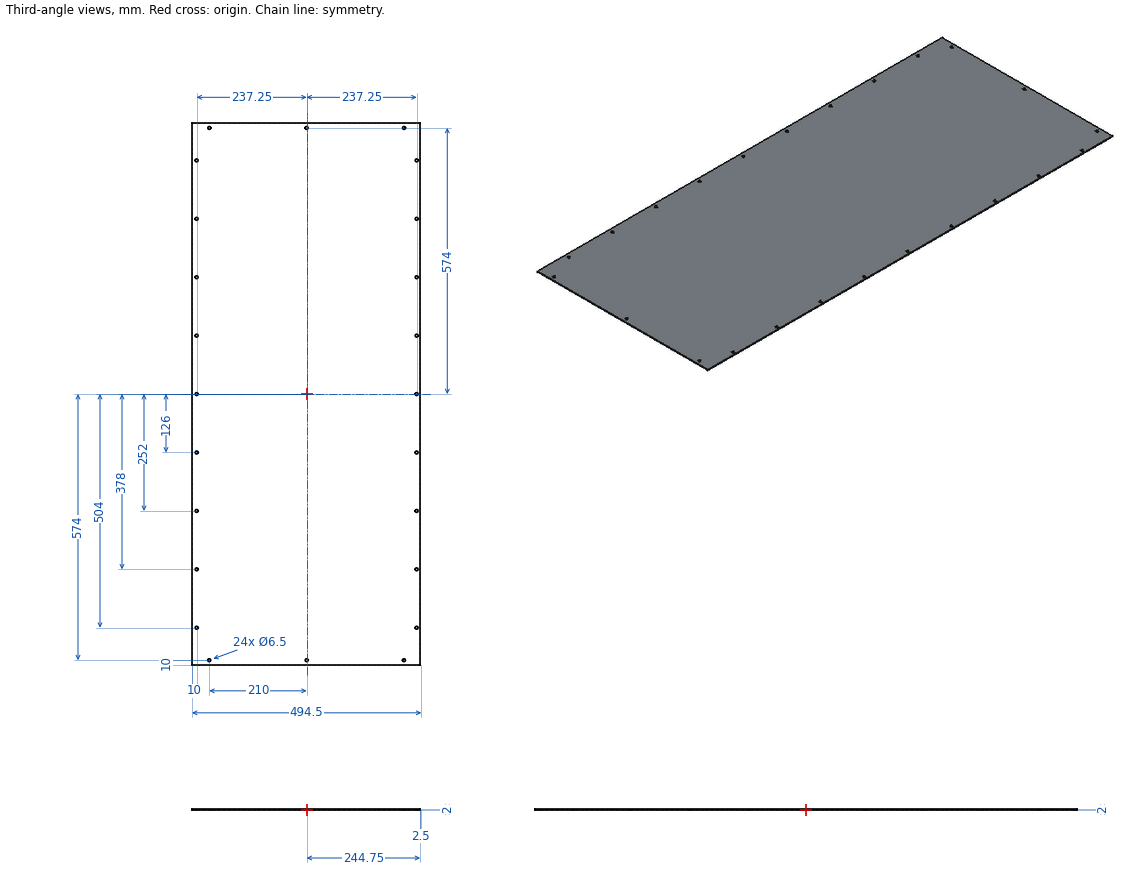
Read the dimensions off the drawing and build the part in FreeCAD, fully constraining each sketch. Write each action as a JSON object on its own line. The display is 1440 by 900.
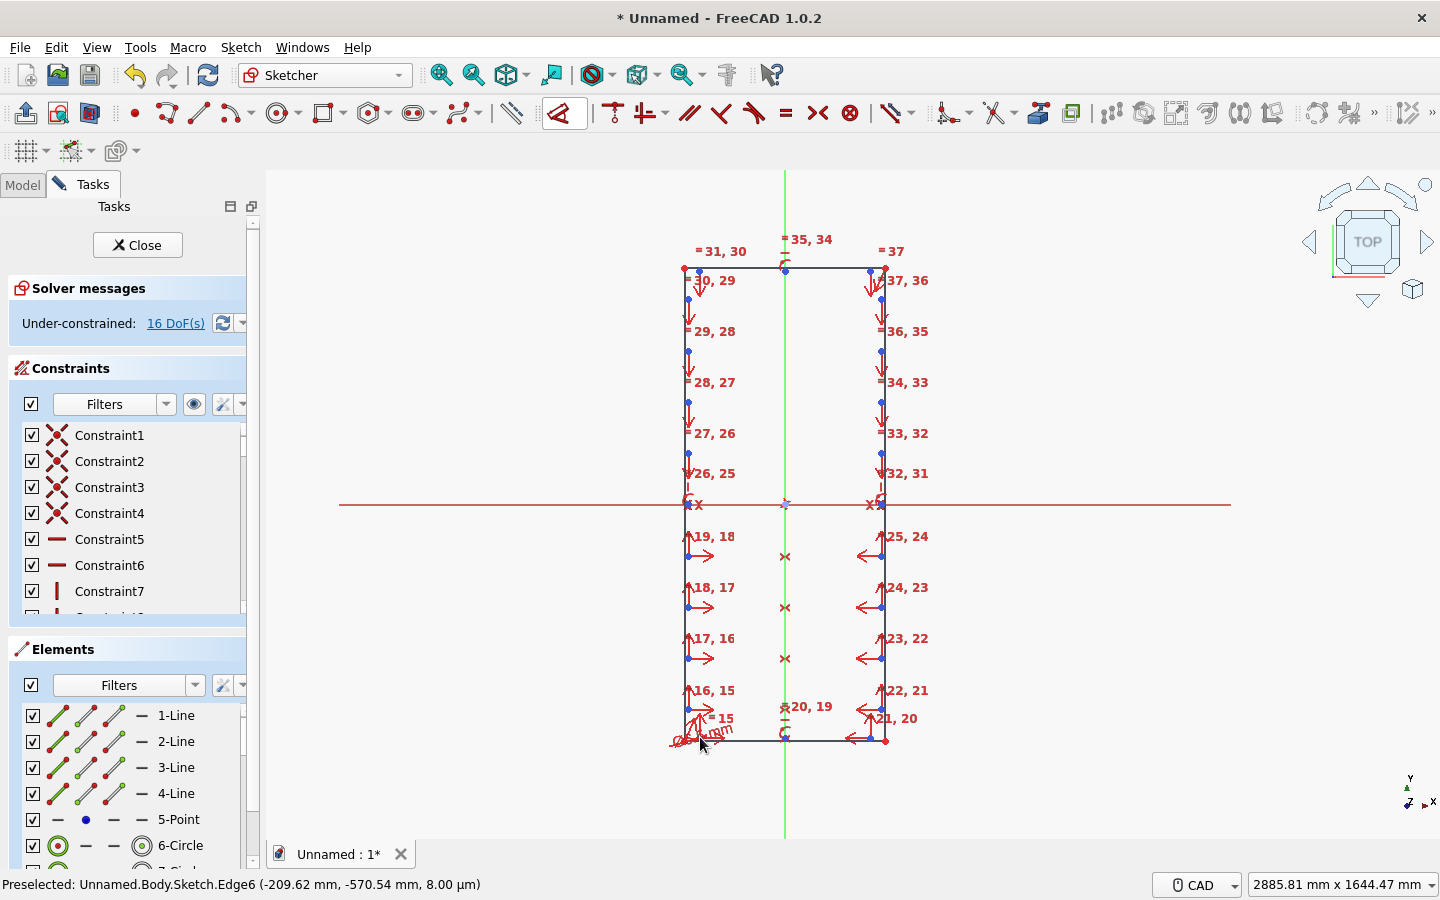
{"action": "left_click", "coordinate": [700, 738]}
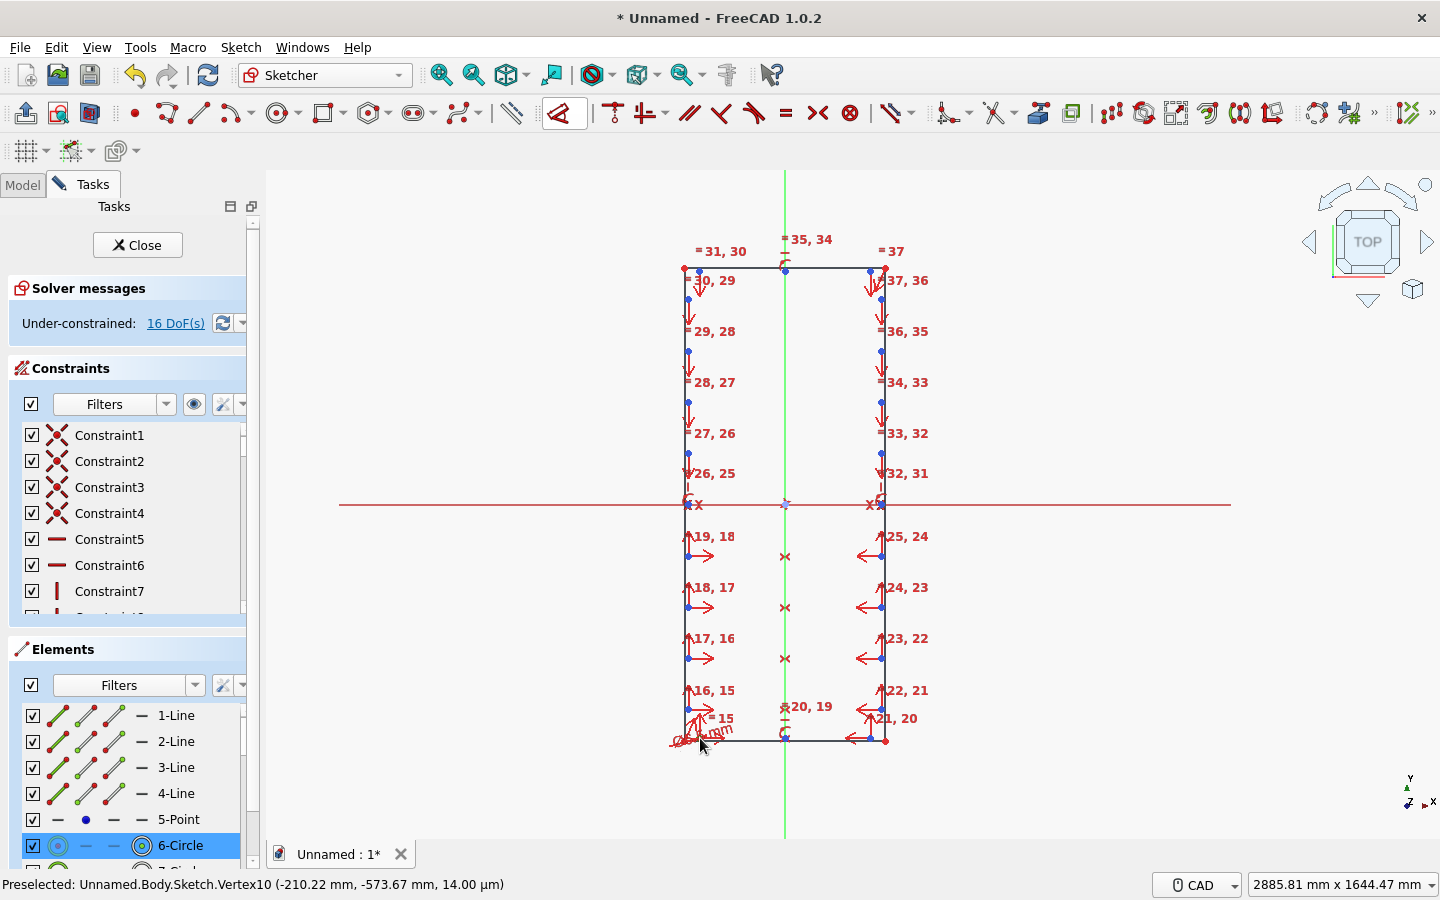
{"action": "key", "text": "l"}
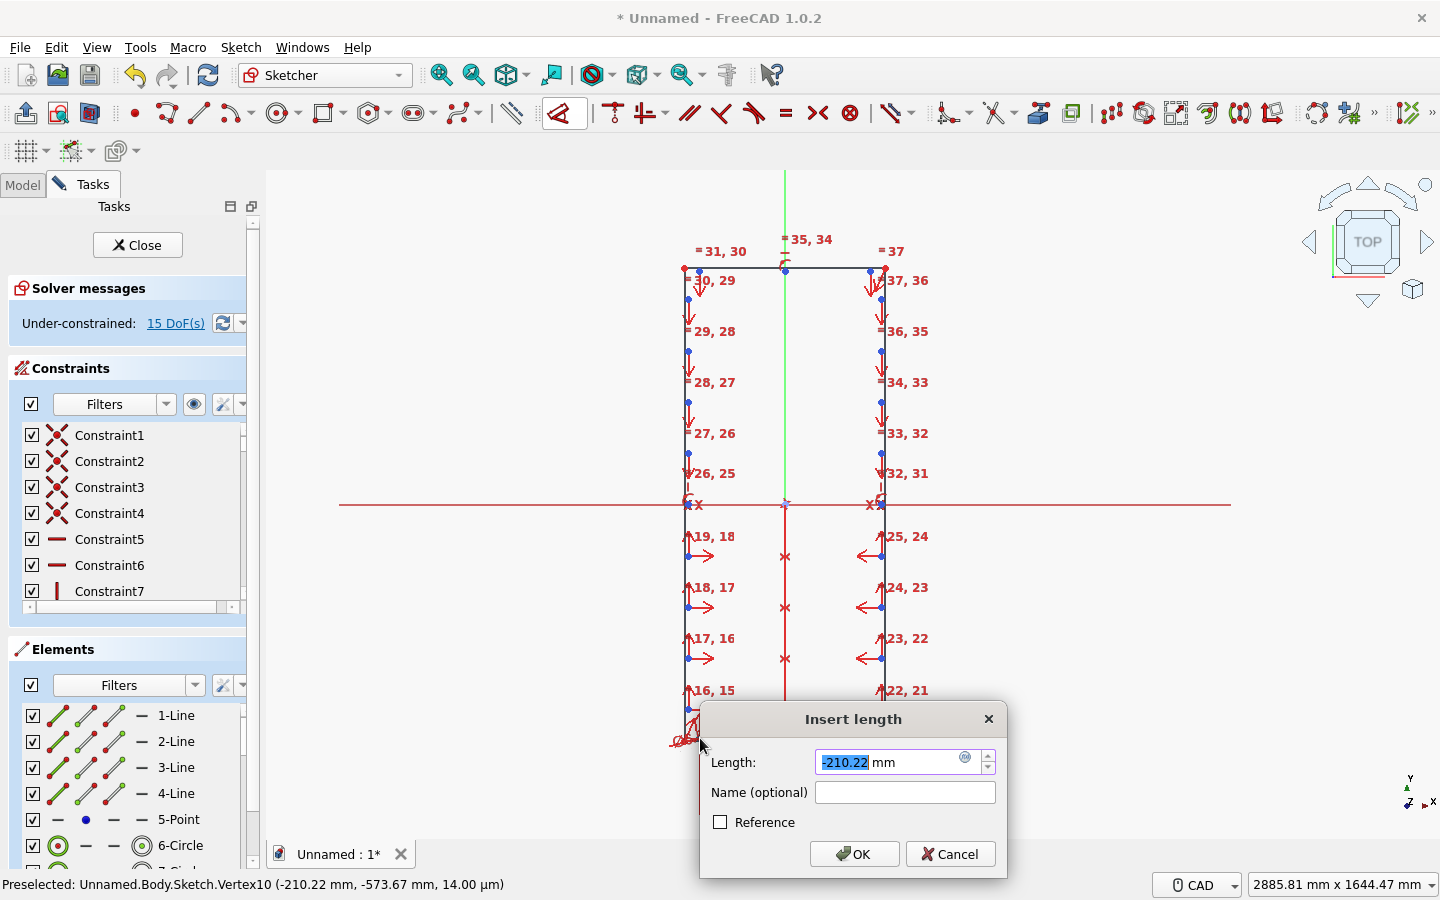
{"action": "type", "text": "-210"}
{"action": "key", "text": "Return"}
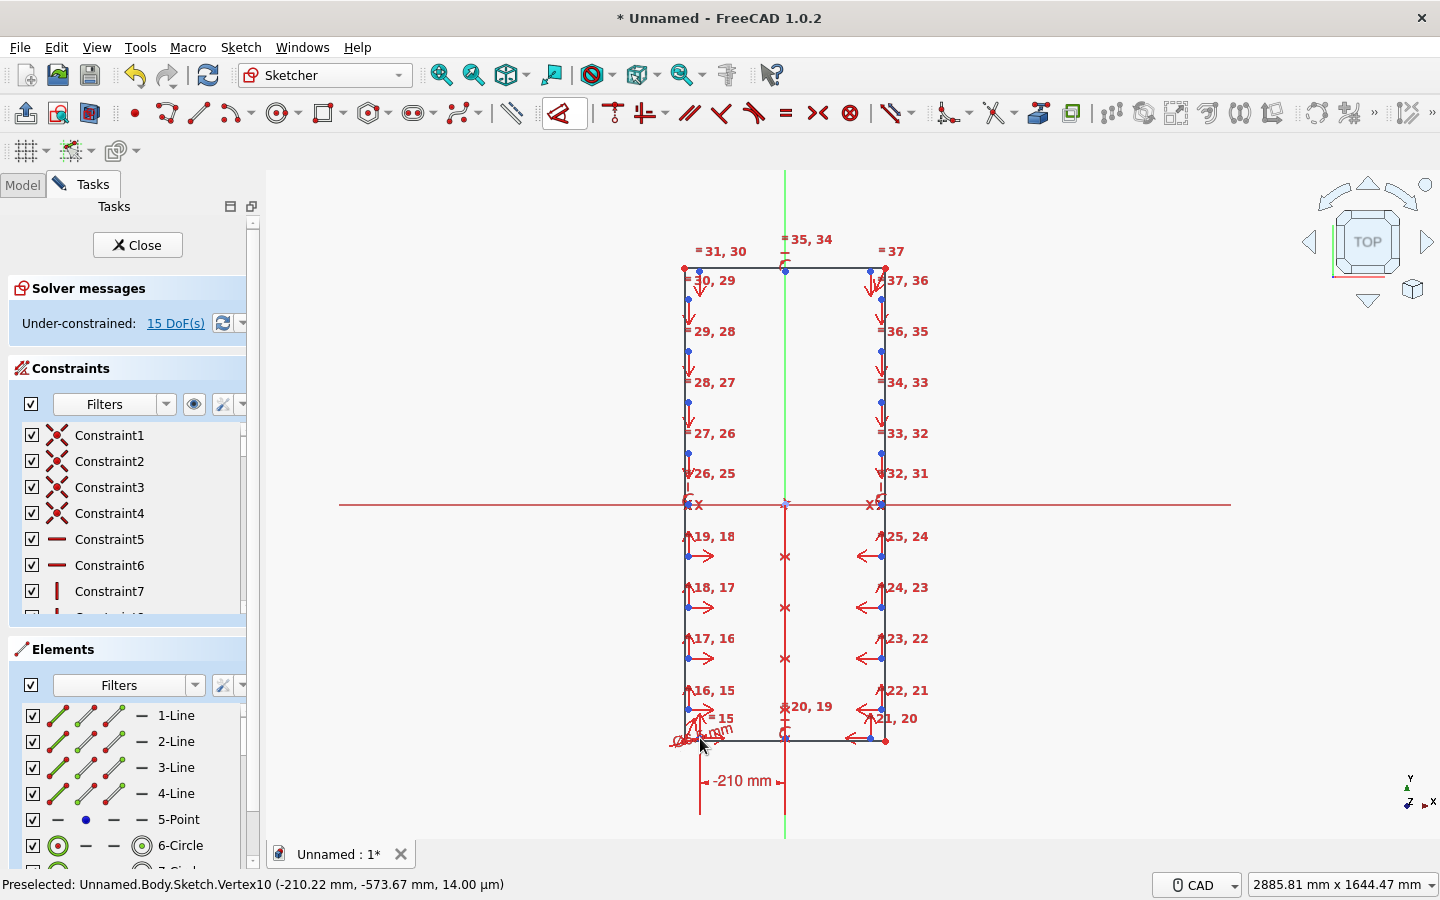
{"action": "left_click", "coordinate": [700, 738]}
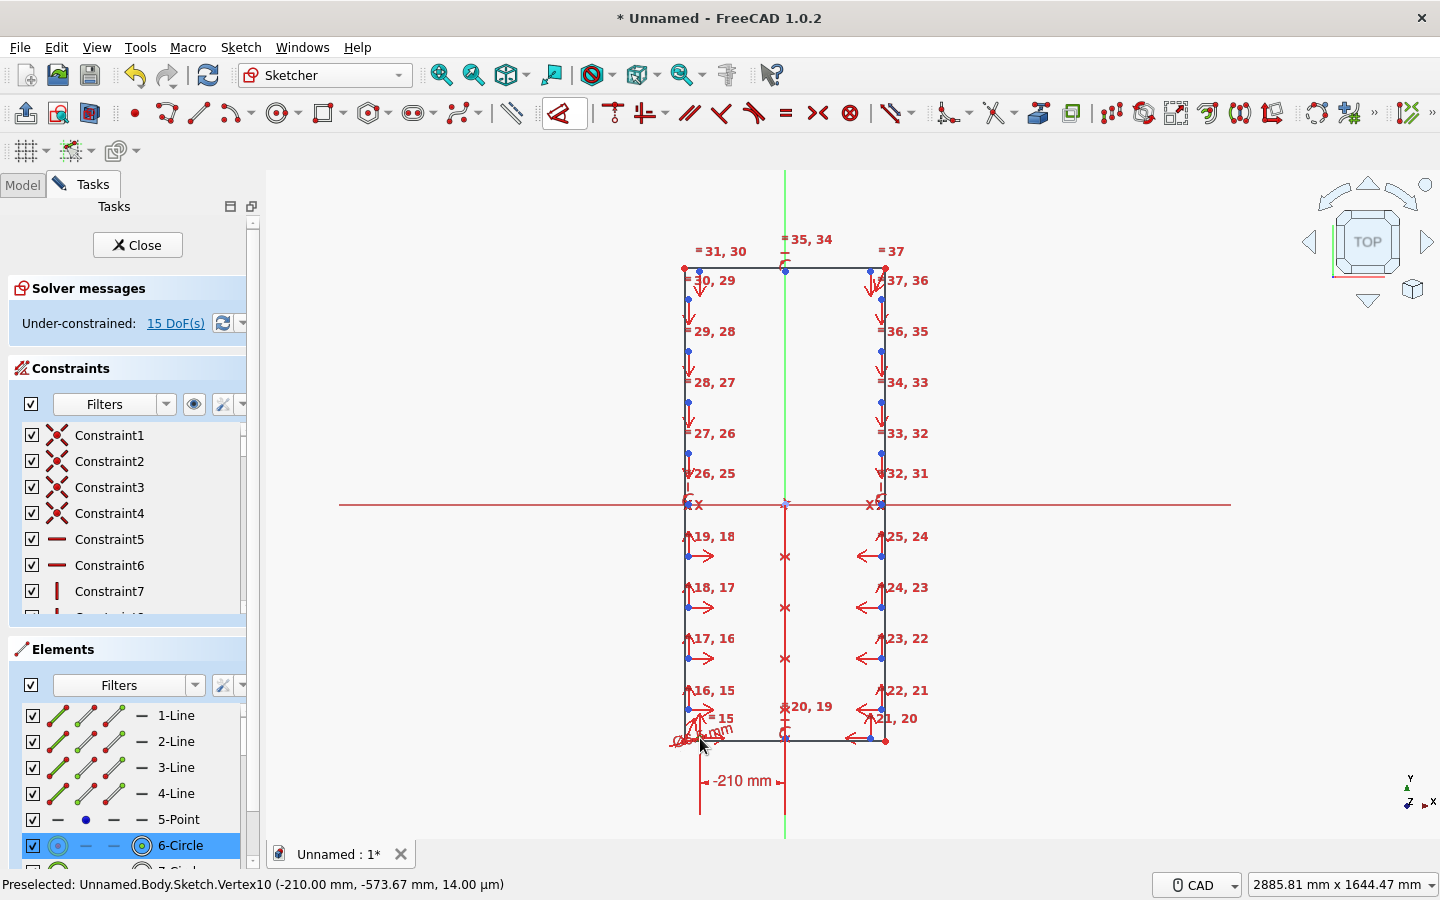
{"action": "key", "text": "i"}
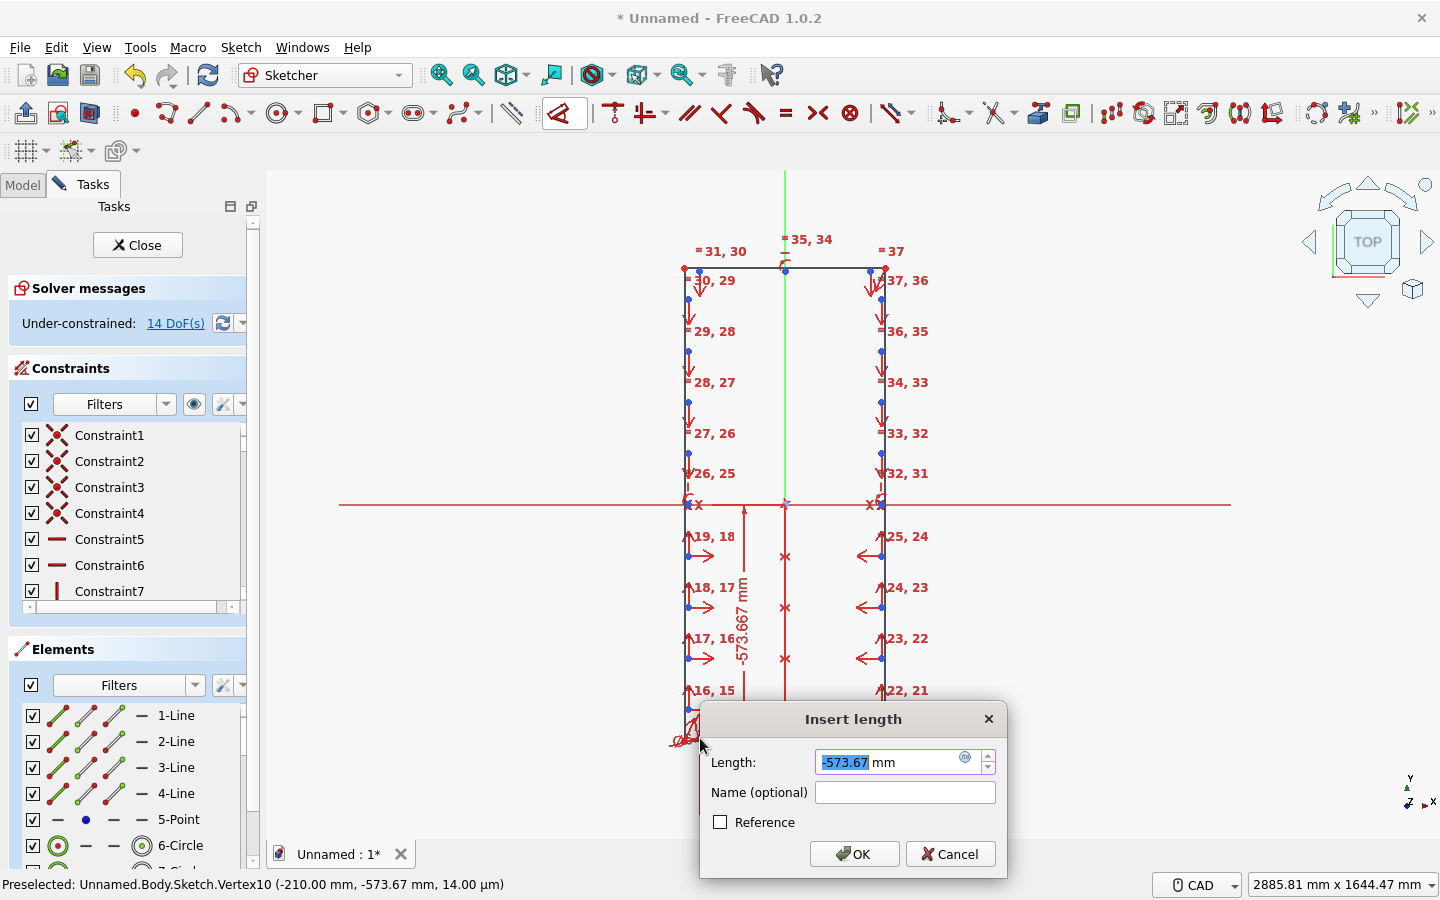
{"action": "type", "text": "-574"}
{"action": "key", "text": "Return"}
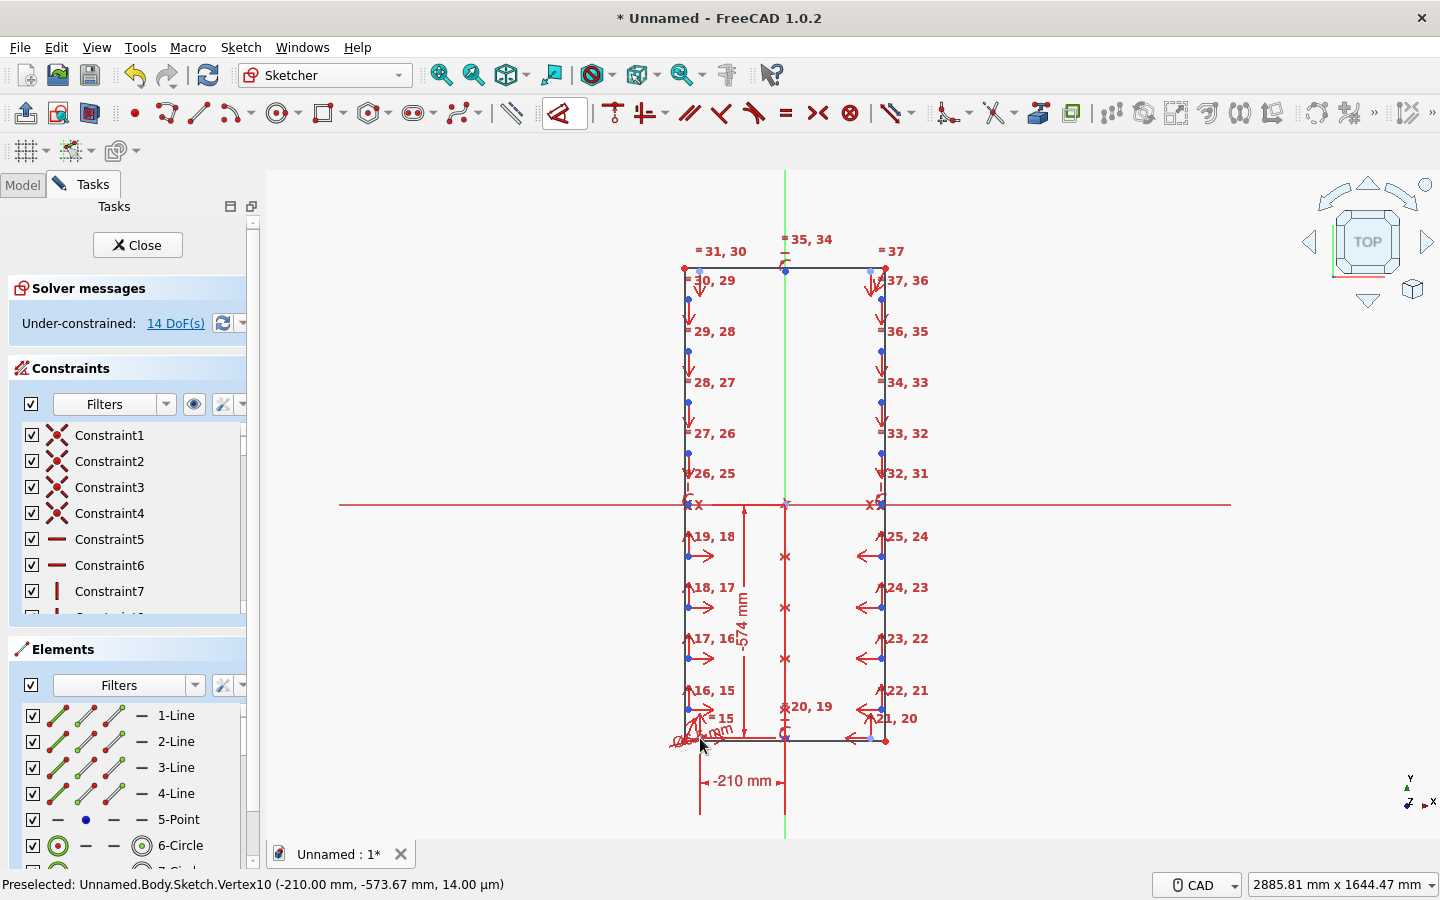
{"action": "left_click", "coordinate": [689, 710]}